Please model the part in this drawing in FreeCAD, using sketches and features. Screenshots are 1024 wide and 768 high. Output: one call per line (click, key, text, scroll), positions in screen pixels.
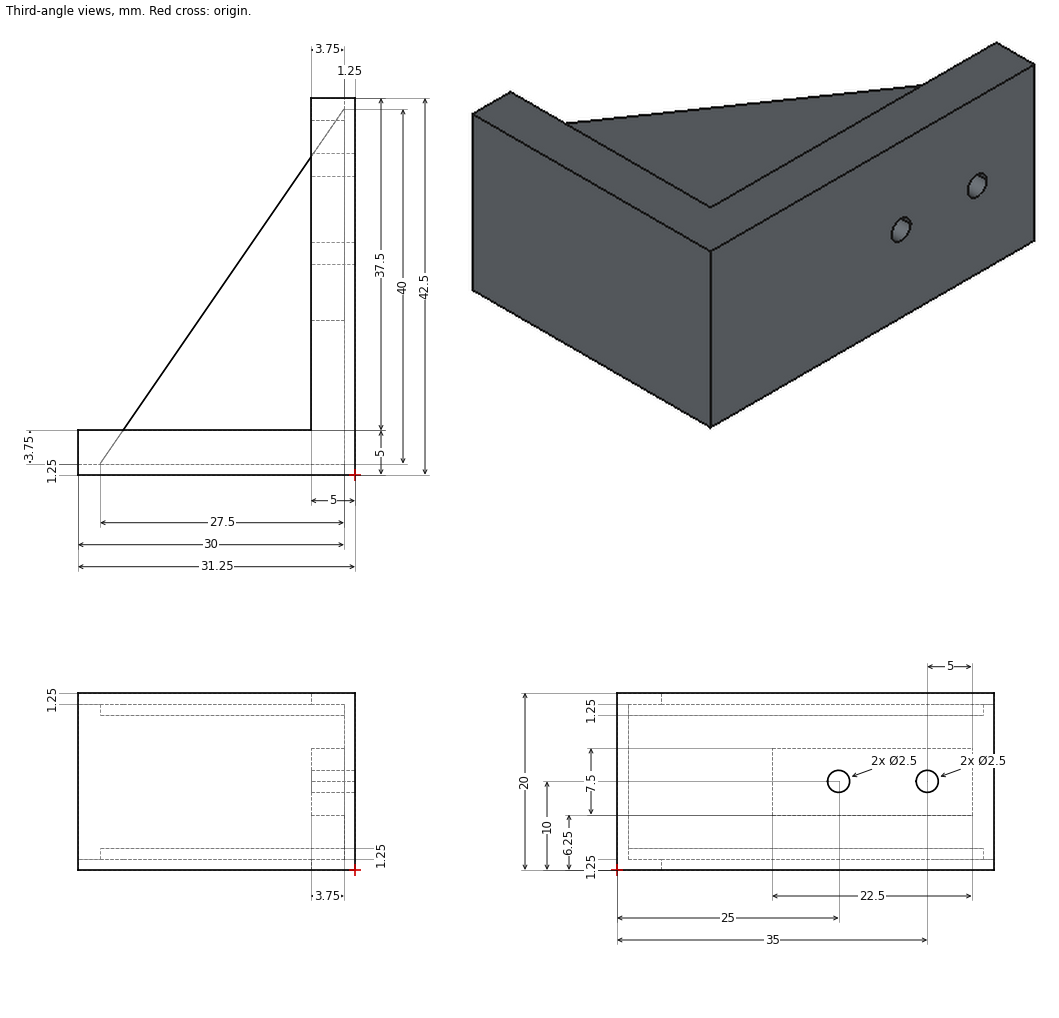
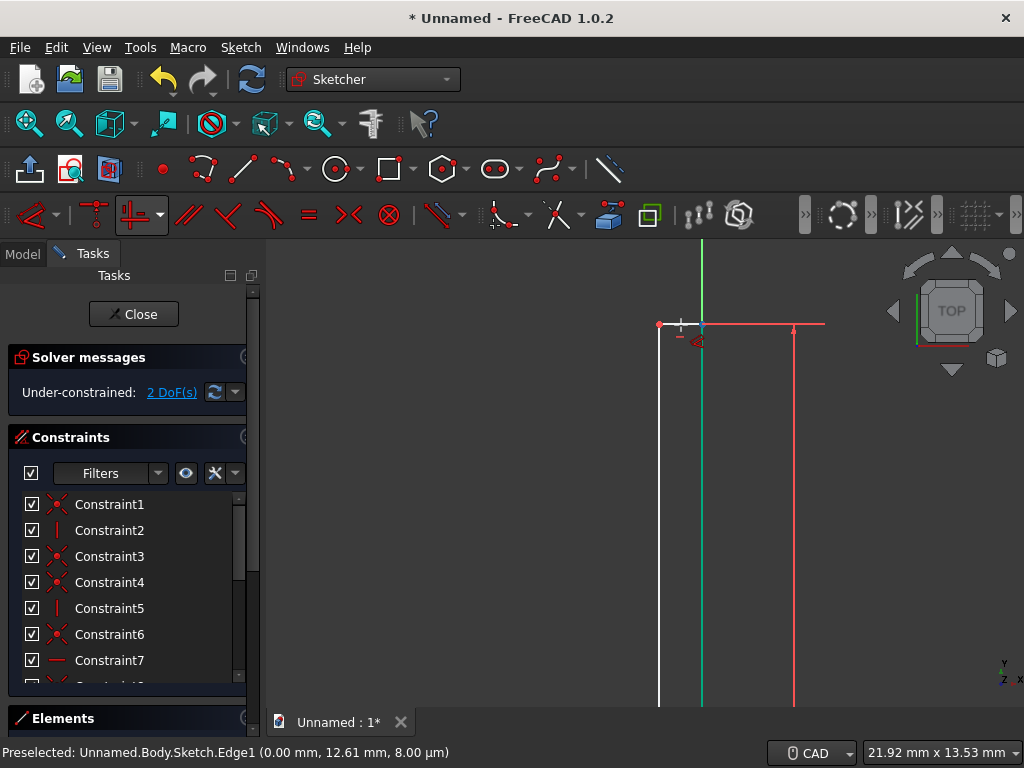
click(681, 324)
click(681, 290)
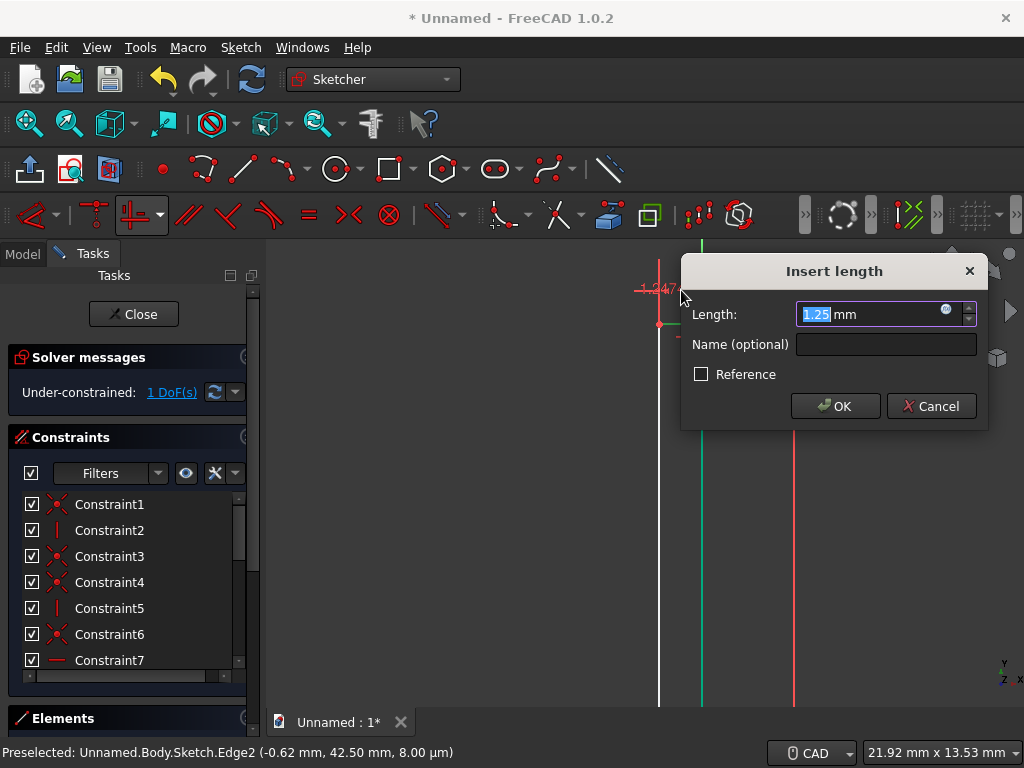
text(1.25)
key(Return)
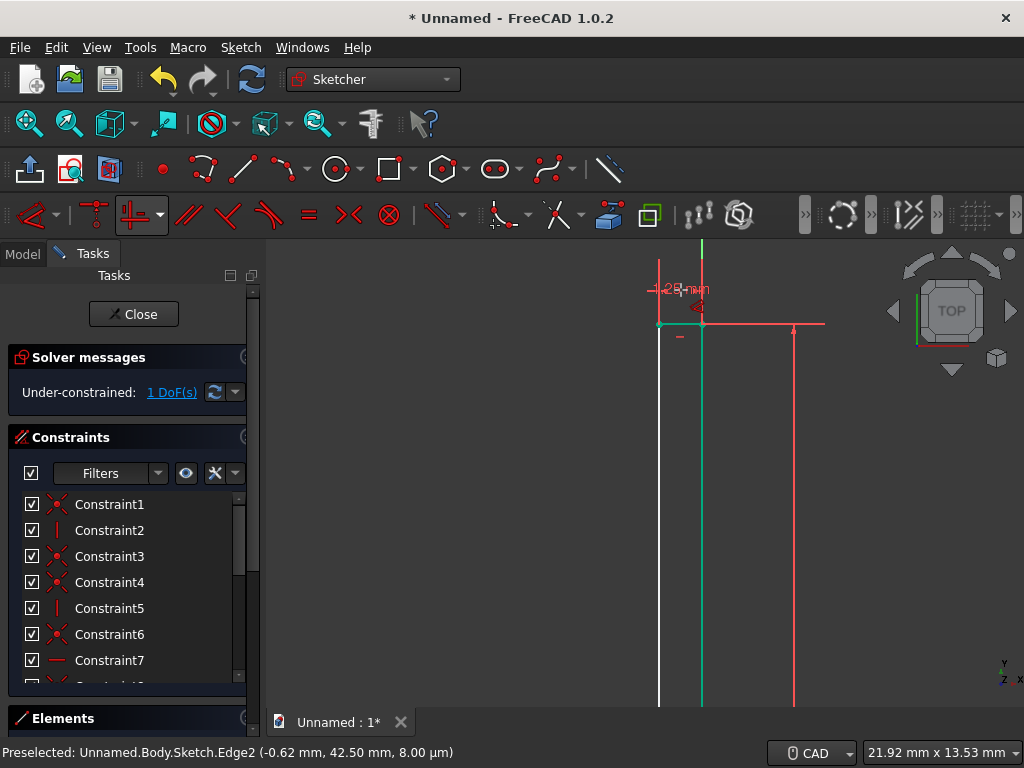
scroll(681, 325, down, 8)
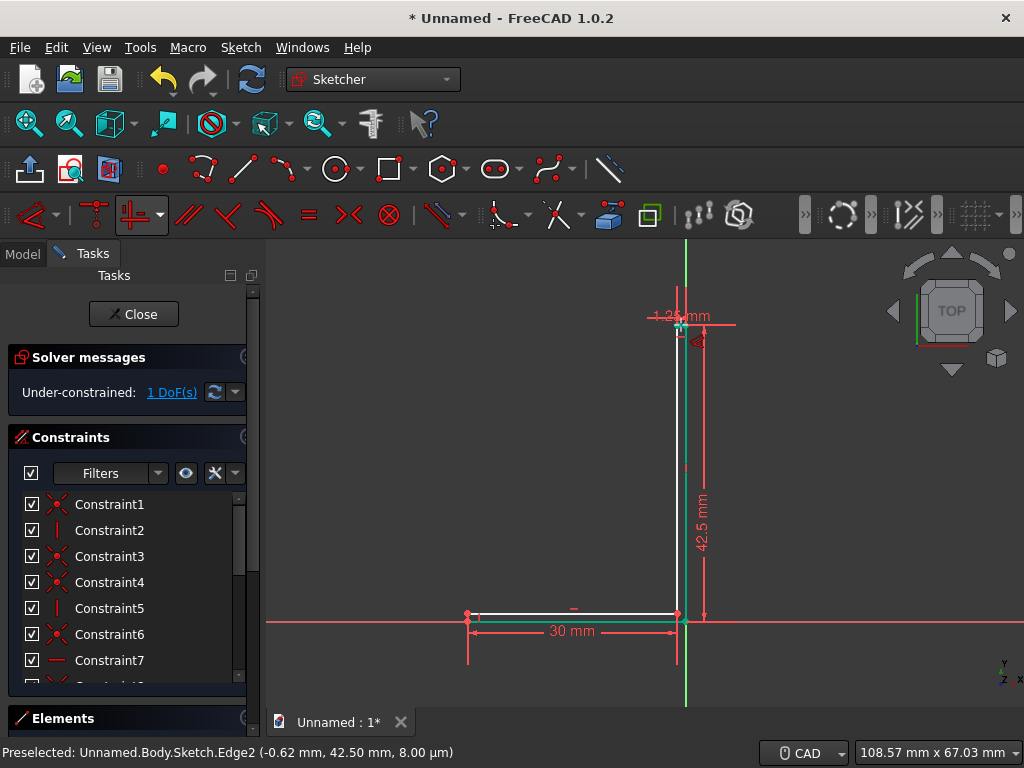
scroll(468, 616, up, 9)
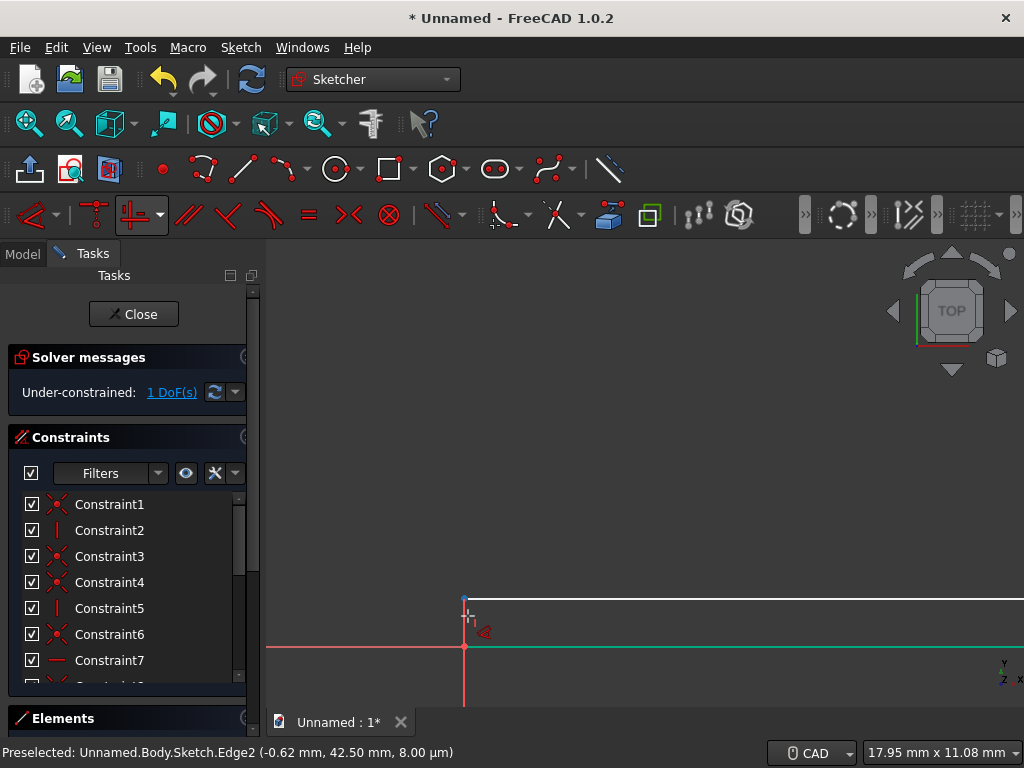
click(464, 613)
click(430, 623)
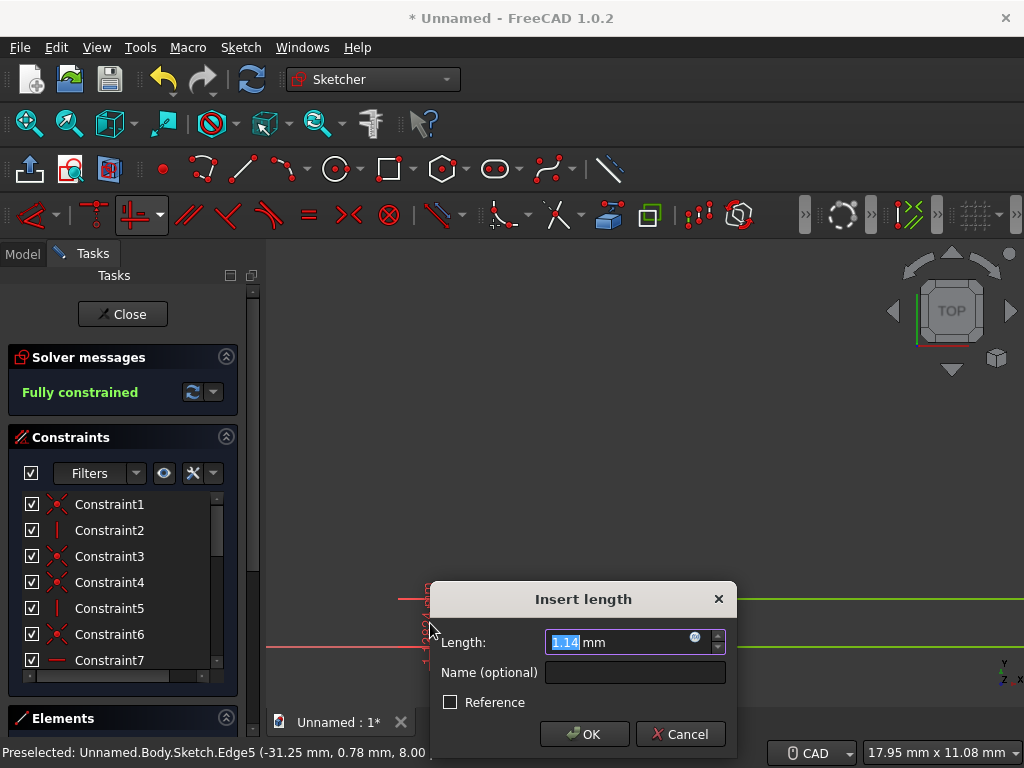
text(1.25)
key(Return)
key(Escape)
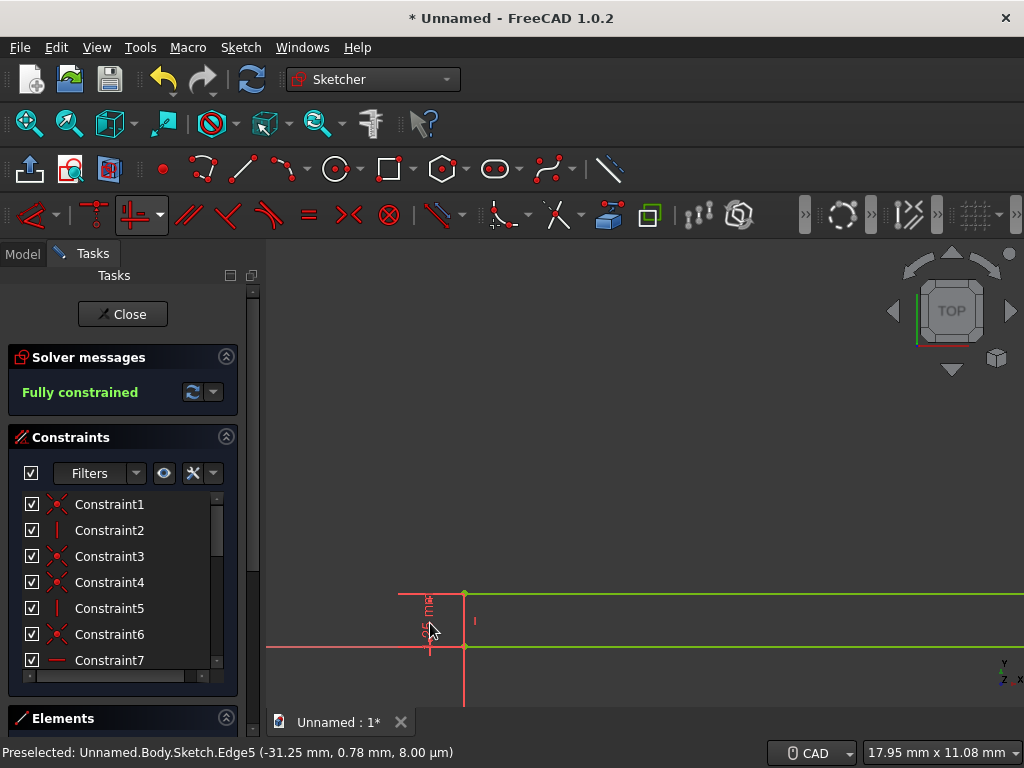
click(123, 314)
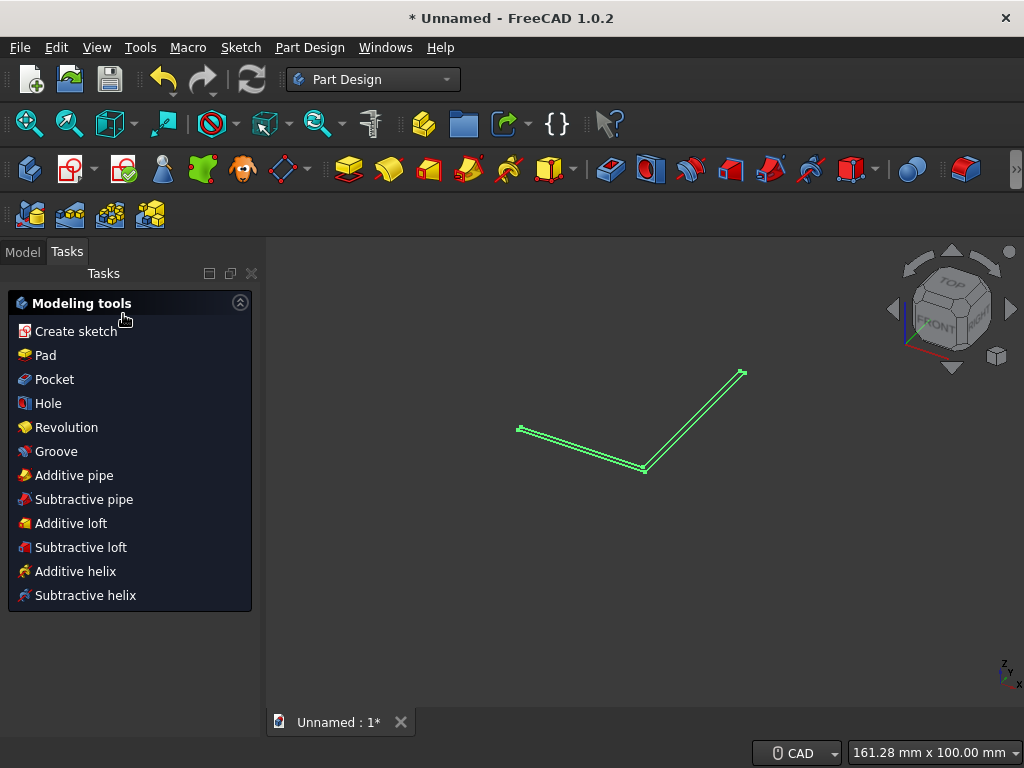
click(350, 170)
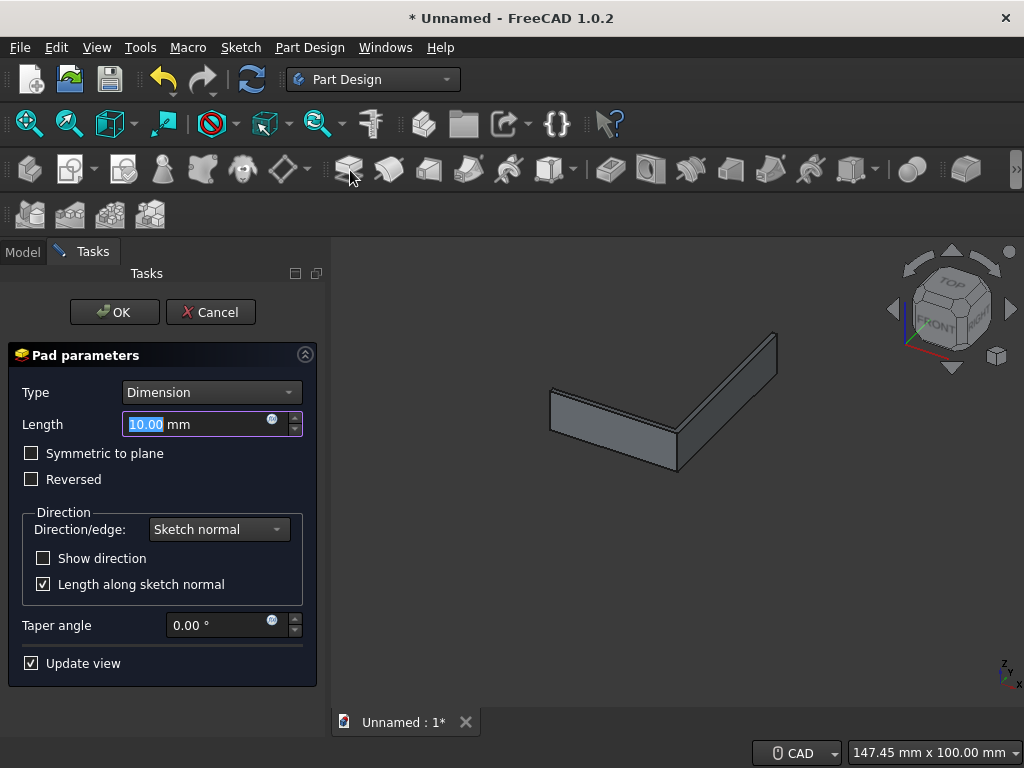
text(20)
key(Tab)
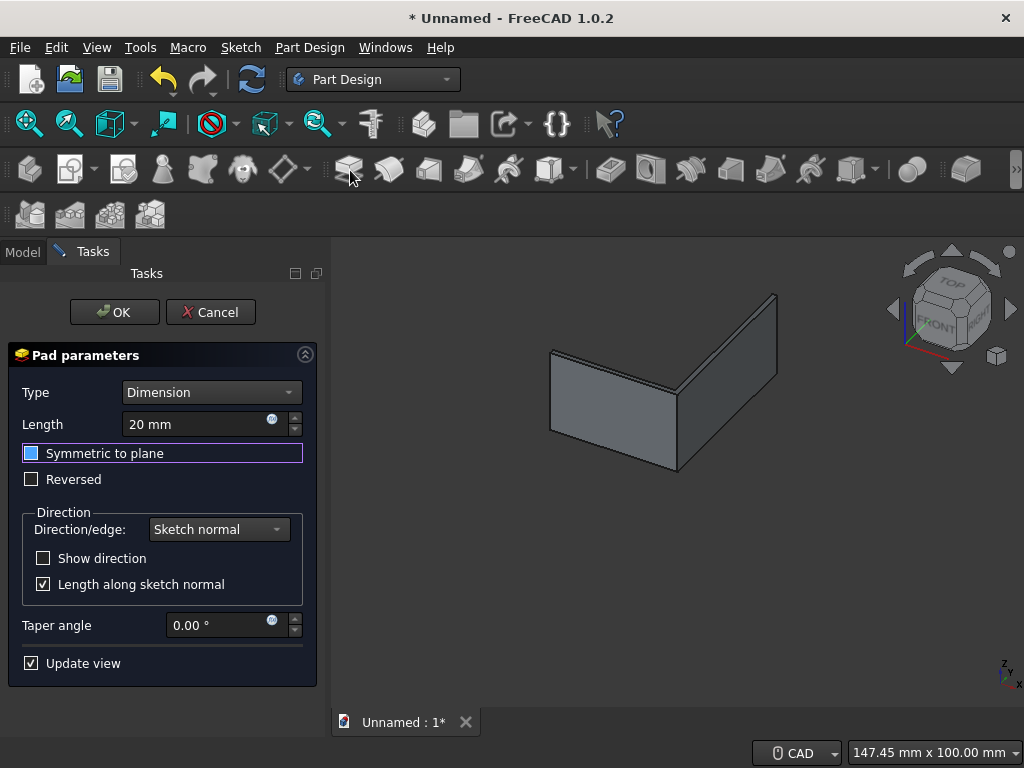
click(115, 312)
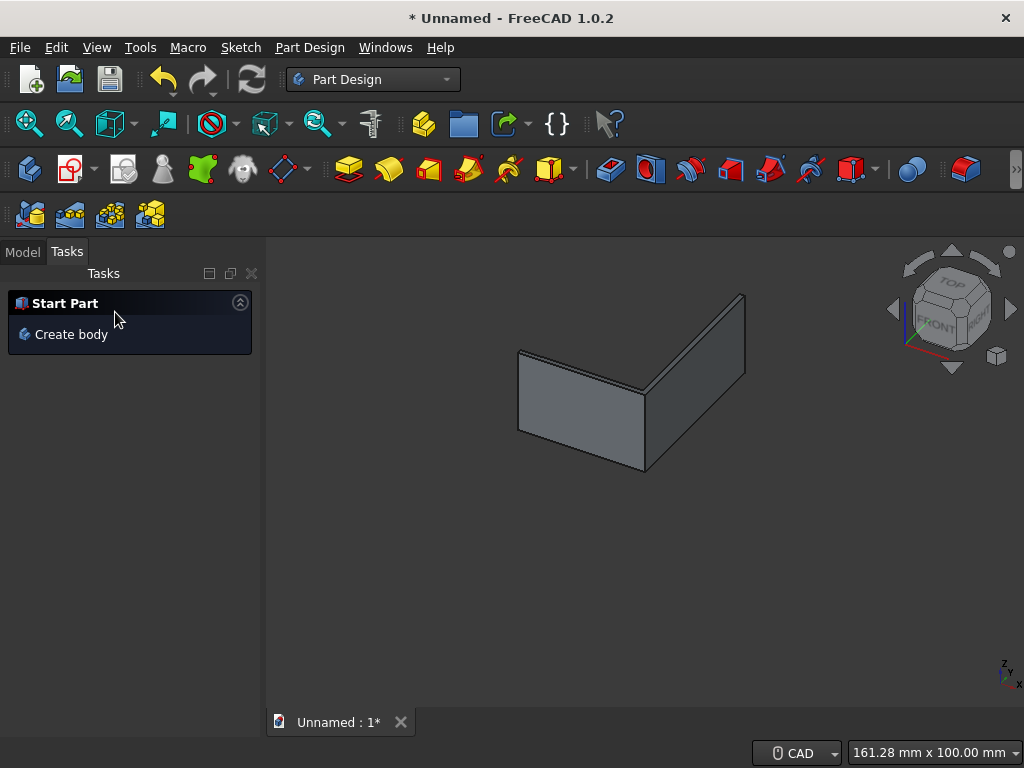
scroll(678, 359, up, 10)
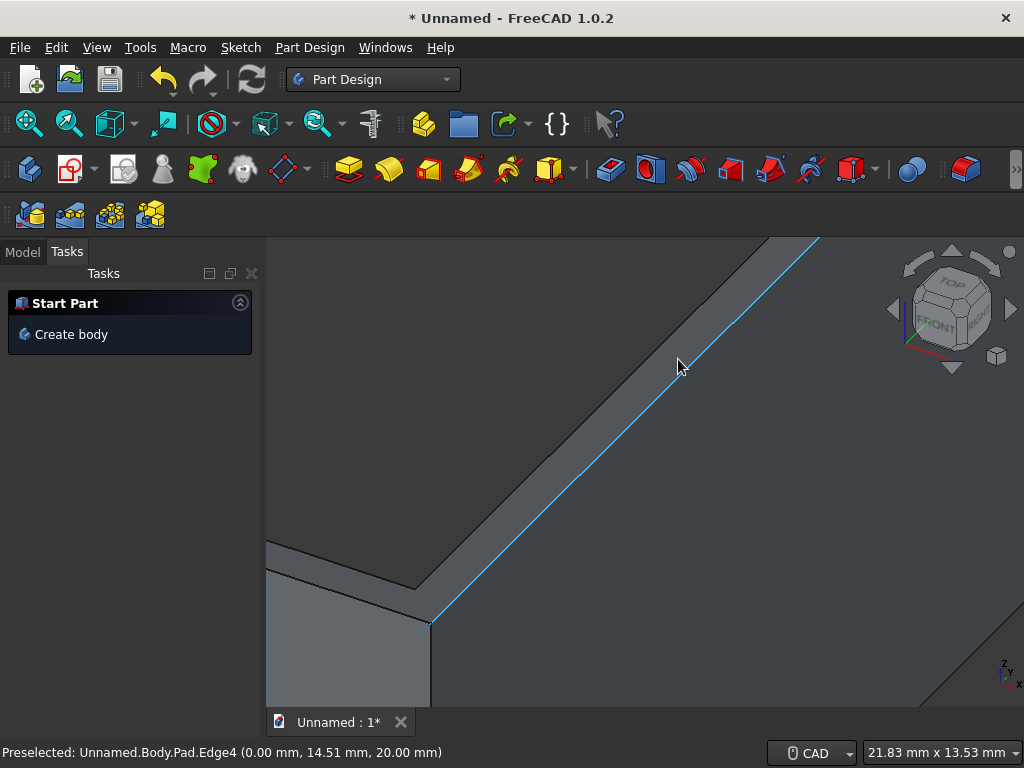
click(671, 367)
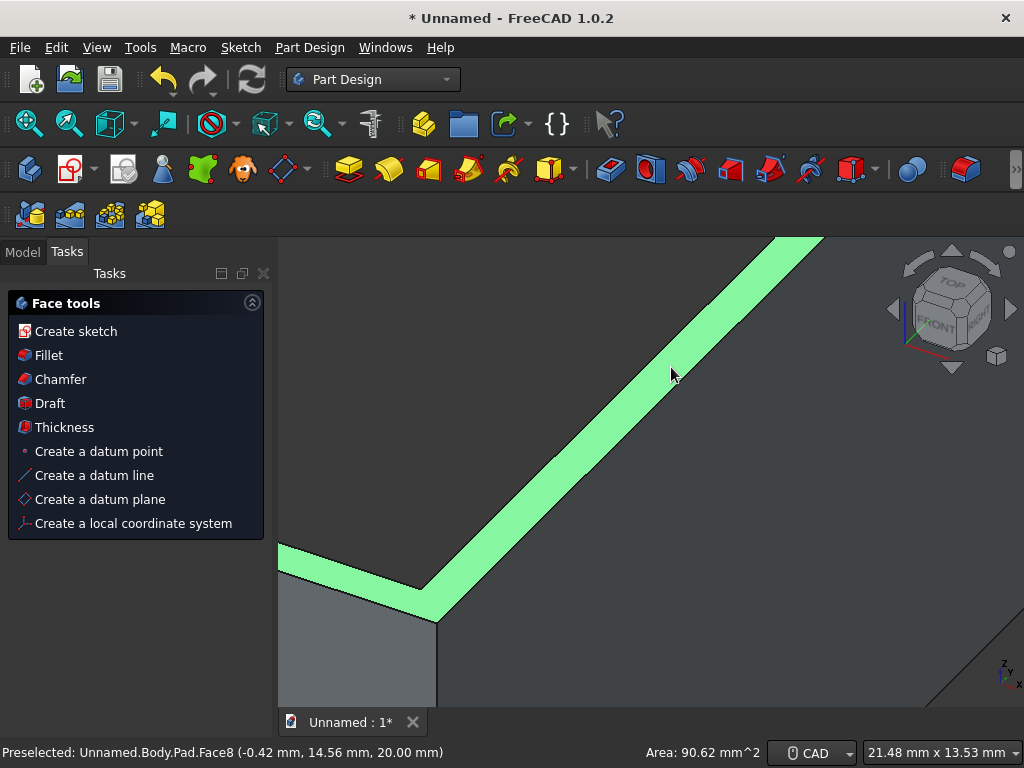
click(70, 170)